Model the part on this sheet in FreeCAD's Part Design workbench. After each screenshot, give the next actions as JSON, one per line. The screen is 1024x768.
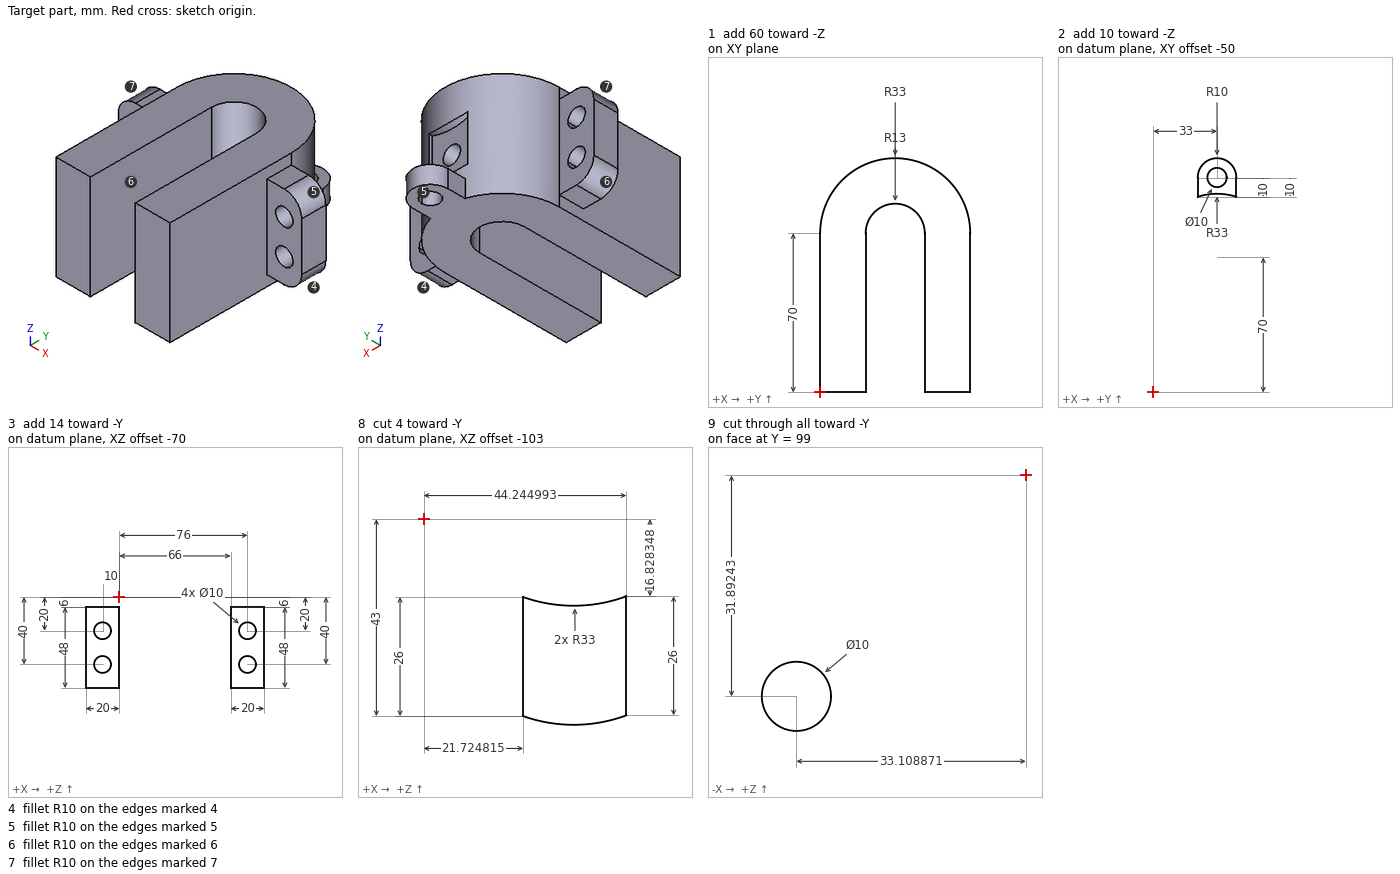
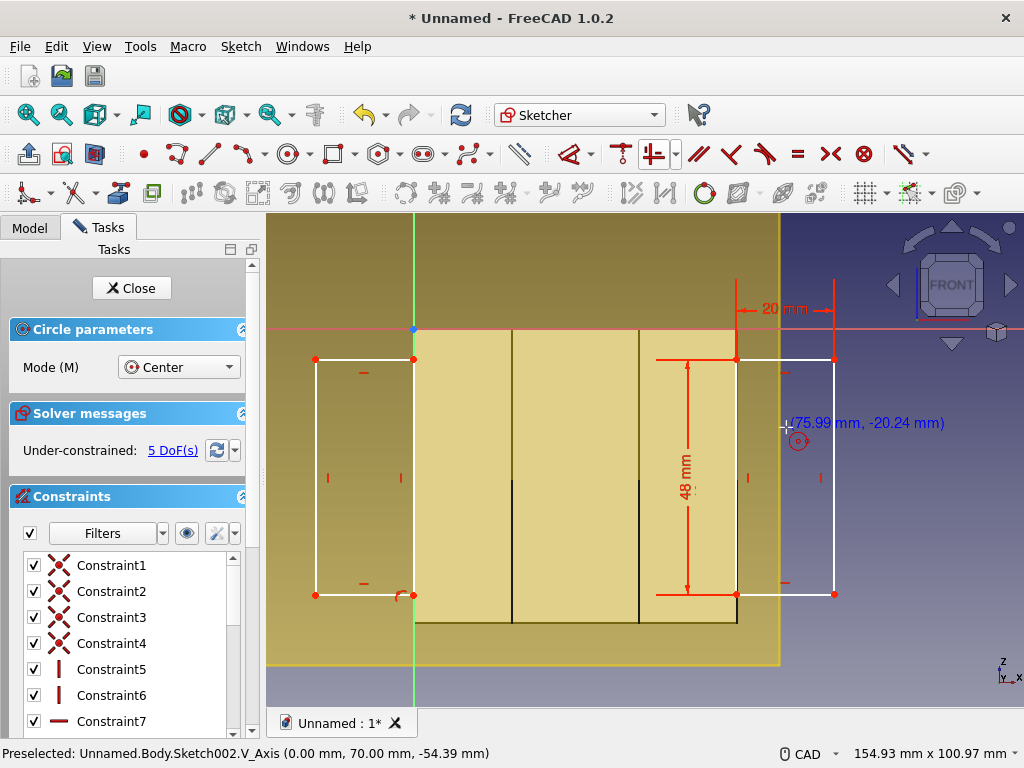
{"action": "left_click", "coordinate": [786, 427]}
{"action": "mouse_move", "coordinate": [803, 410]}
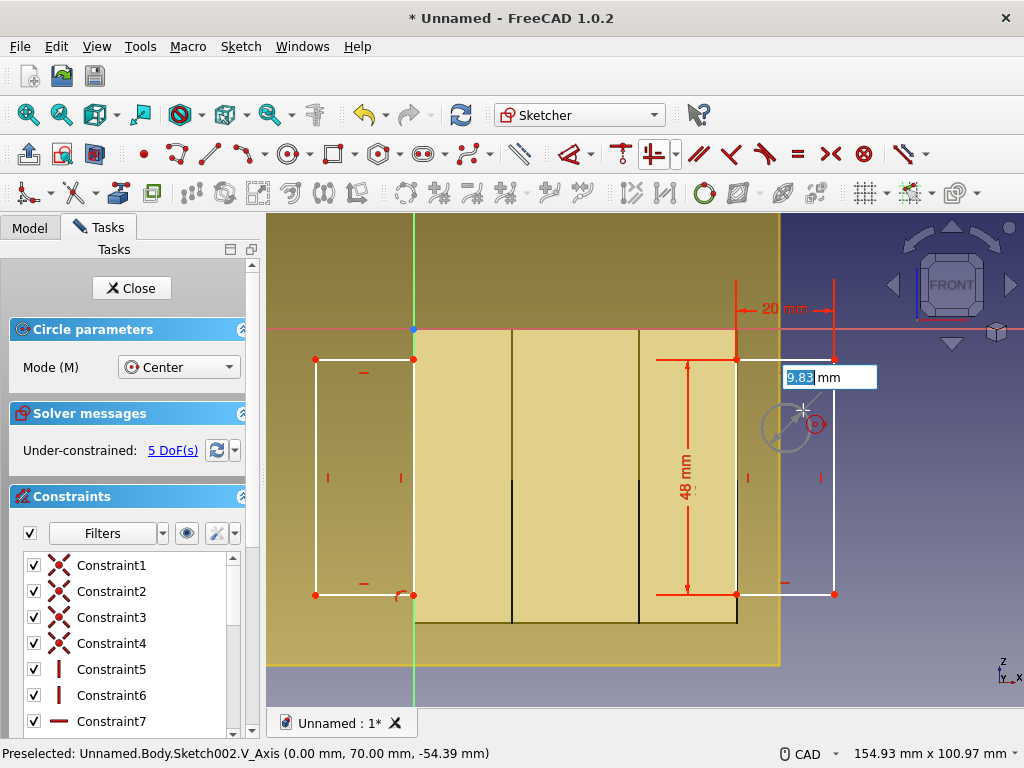
{"action": "type", "text": "10"}
{"action": "key", "text": "Return"}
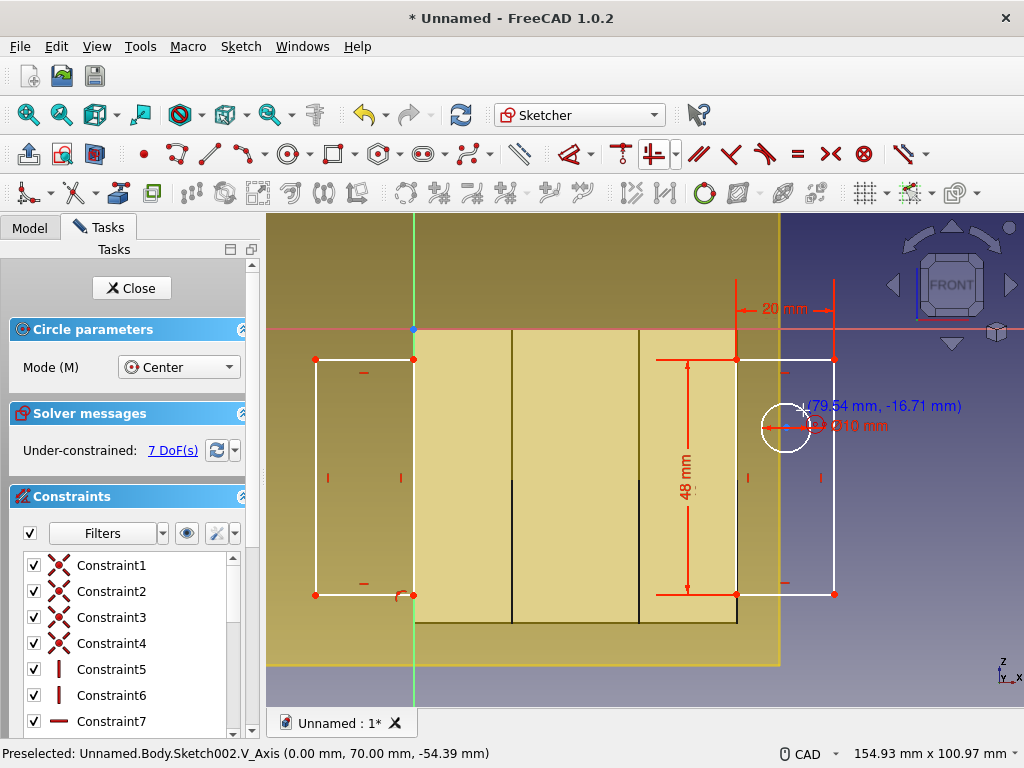
{"action": "left_click", "coordinate": [786, 525]}
{"action": "mouse_move", "coordinate": [803, 508]}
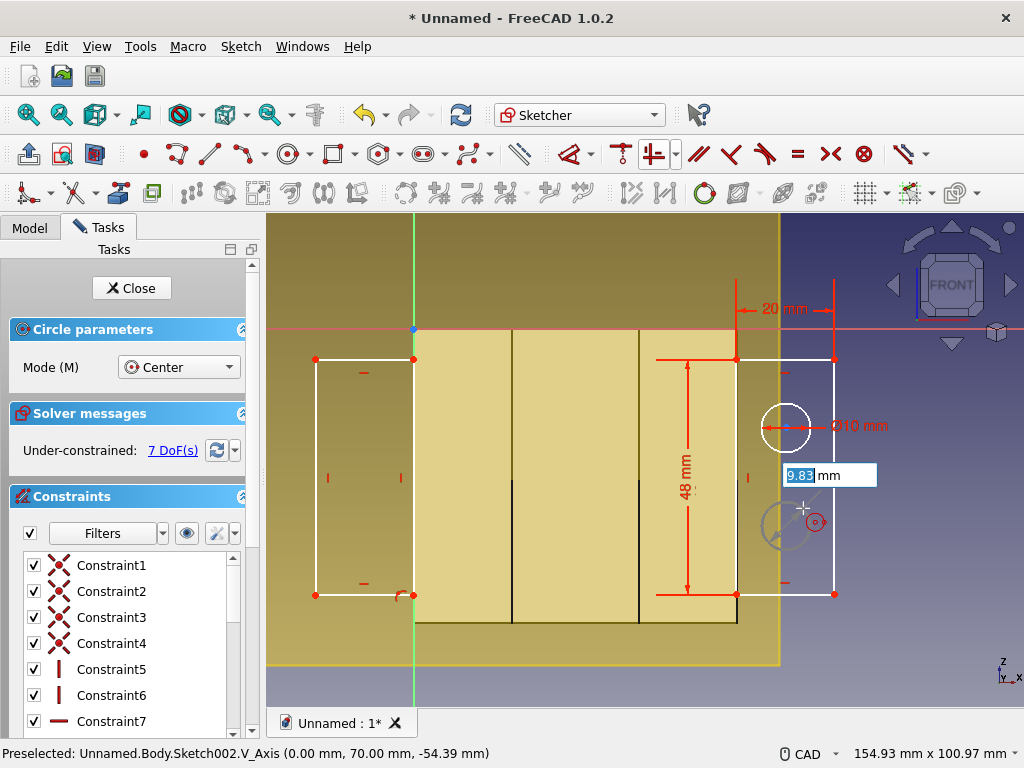
{"action": "type", "text": "10"}
{"action": "key", "text": "Return"}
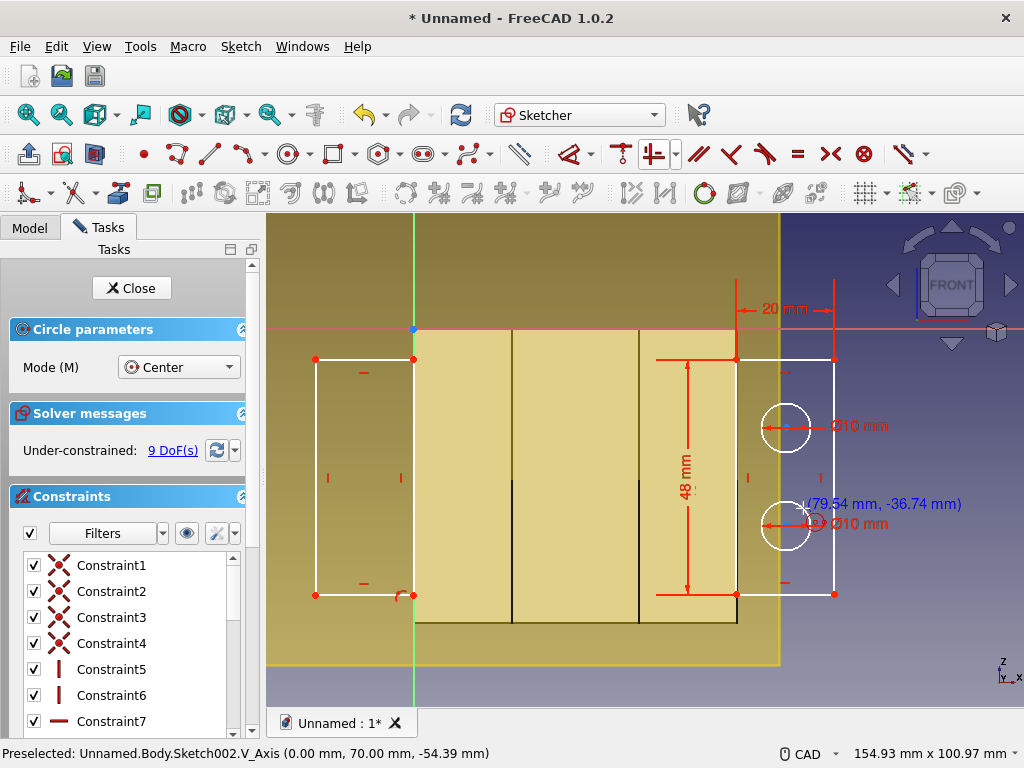
{"action": "left_click", "coordinate": [365, 427]}
{"action": "mouse_move", "coordinate": [382, 410]}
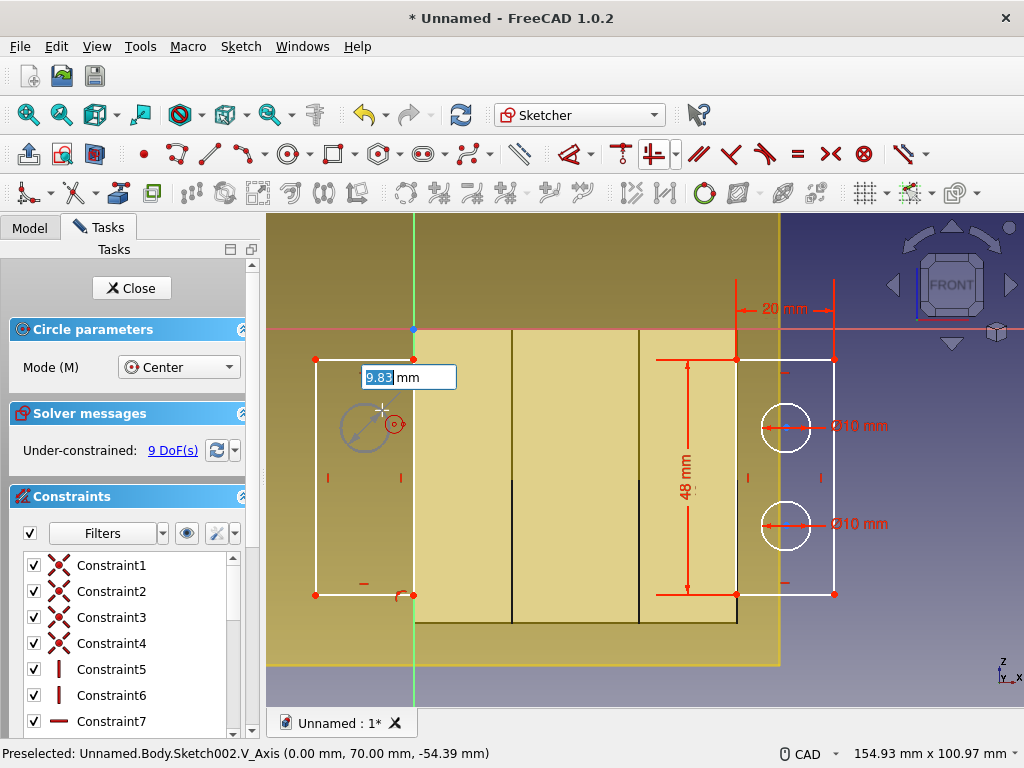
{"action": "type", "text": "10"}
{"action": "key", "text": "Return"}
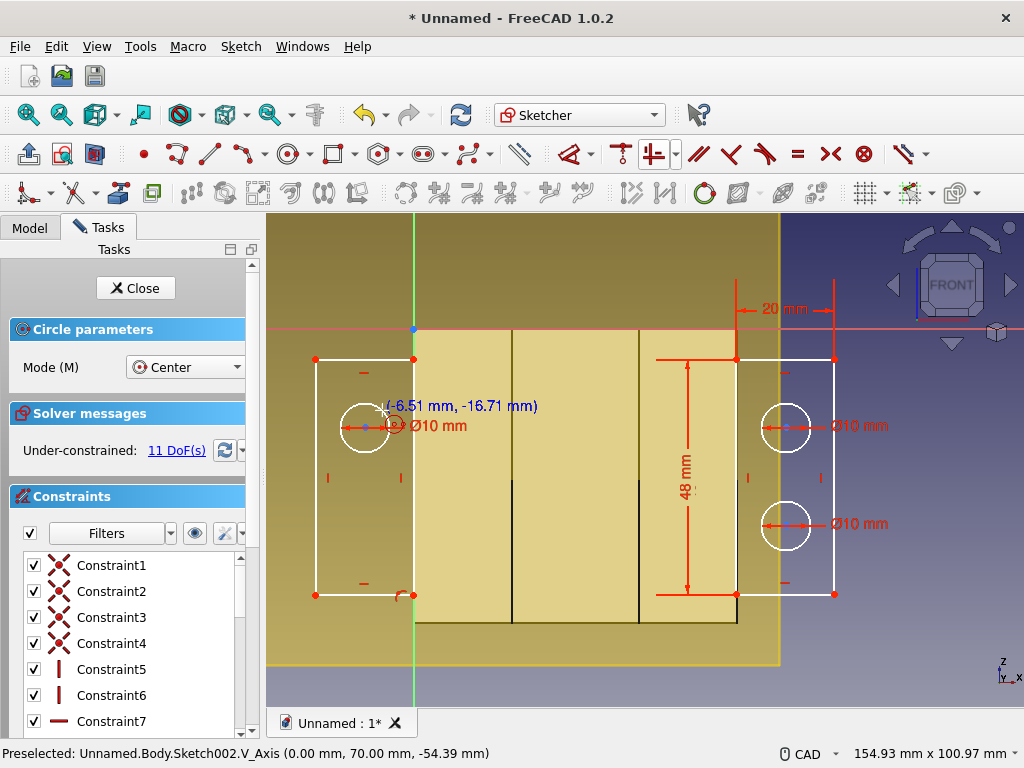
{"action": "left_click", "coordinate": [365, 525]}
{"action": "mouse_move", "coordinate": [382, 508]}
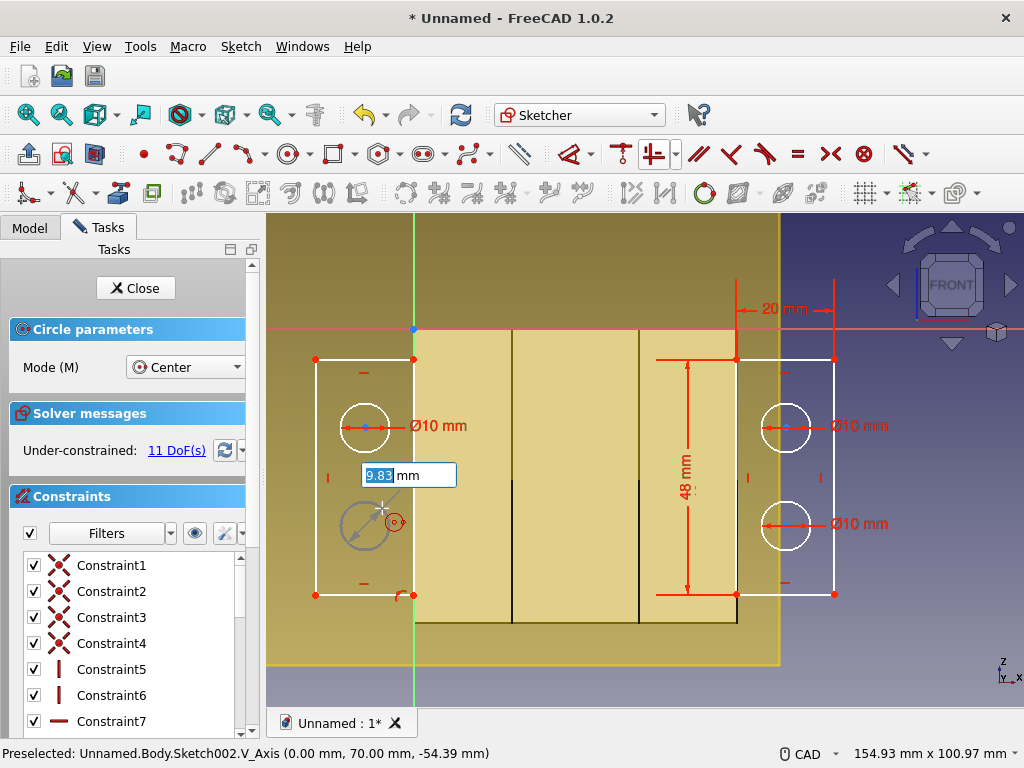
{"action": "type", "text": "10"}
{"action": "key", "text": "Return"}
{"action": "key", "text": "Escape"}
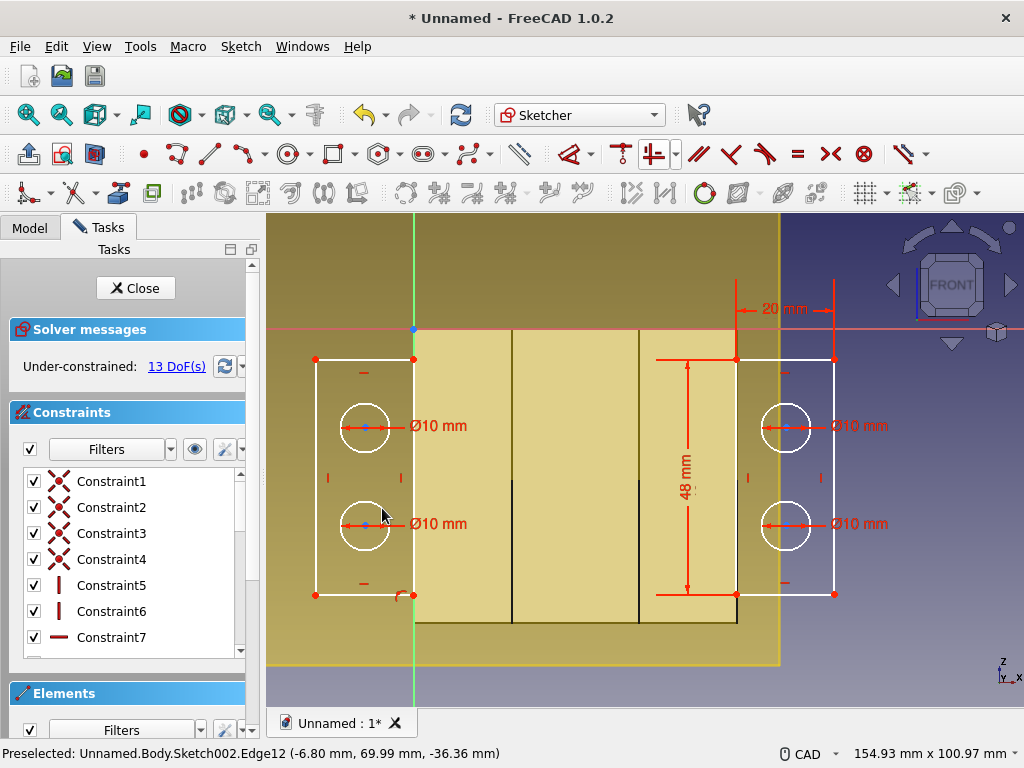
{"action": "left_click", "coordinate": [786, 428]}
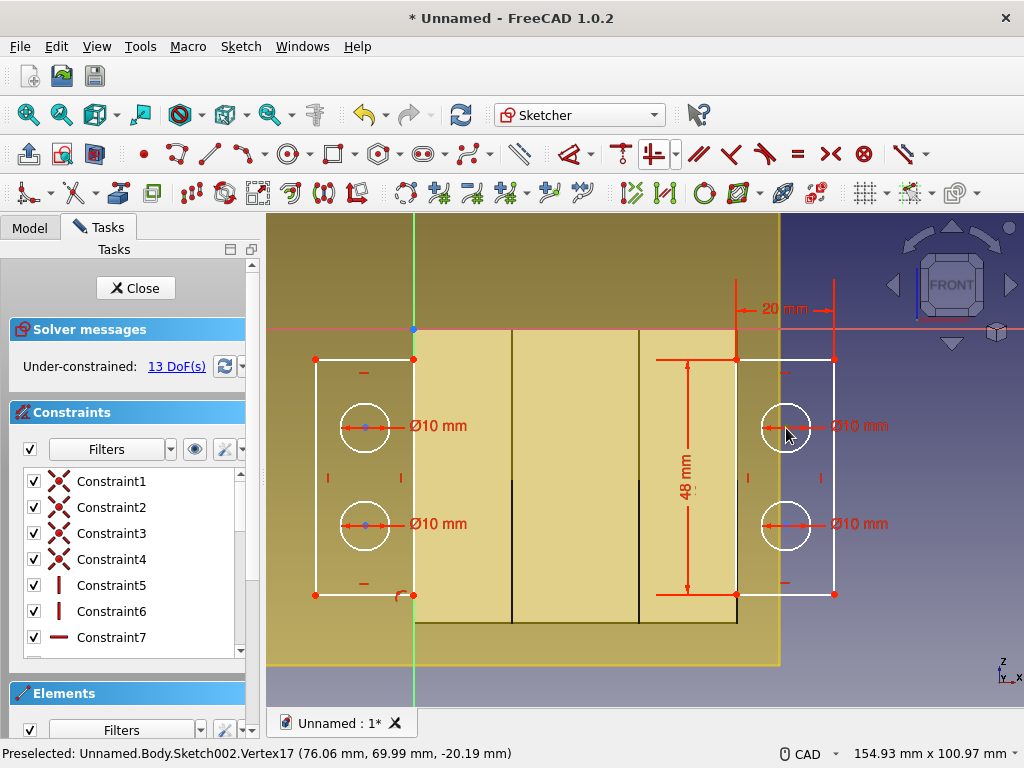
{"action": "left_click", "coordinate": [786, 526]}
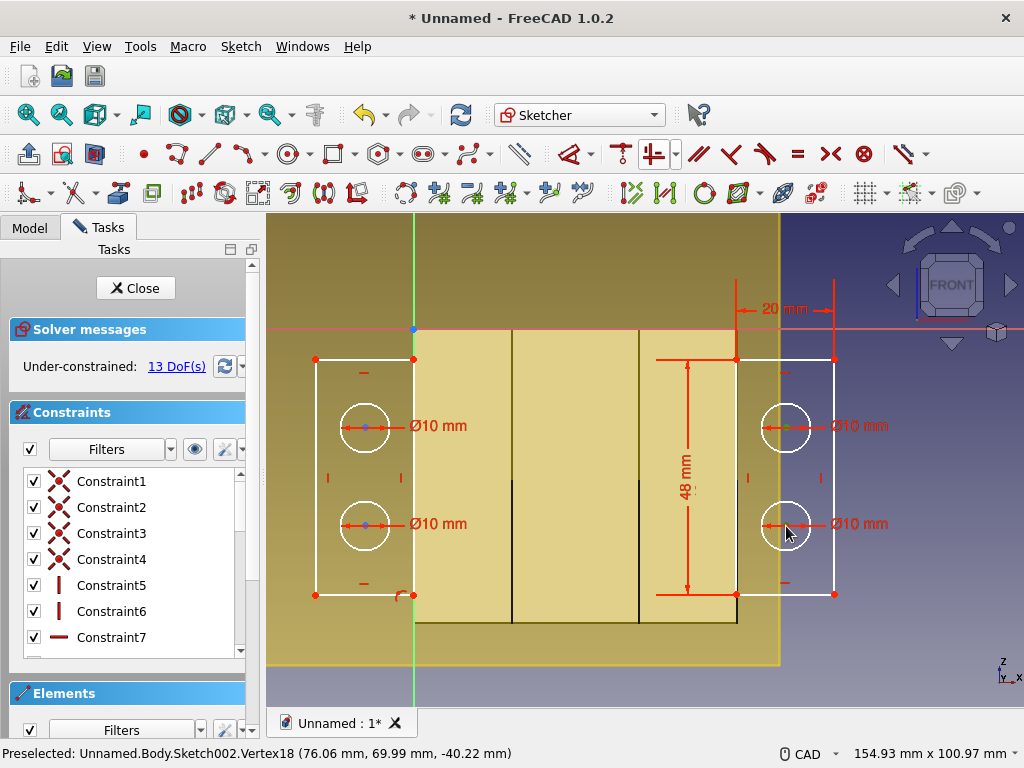
{"action": "key", "text": "v"}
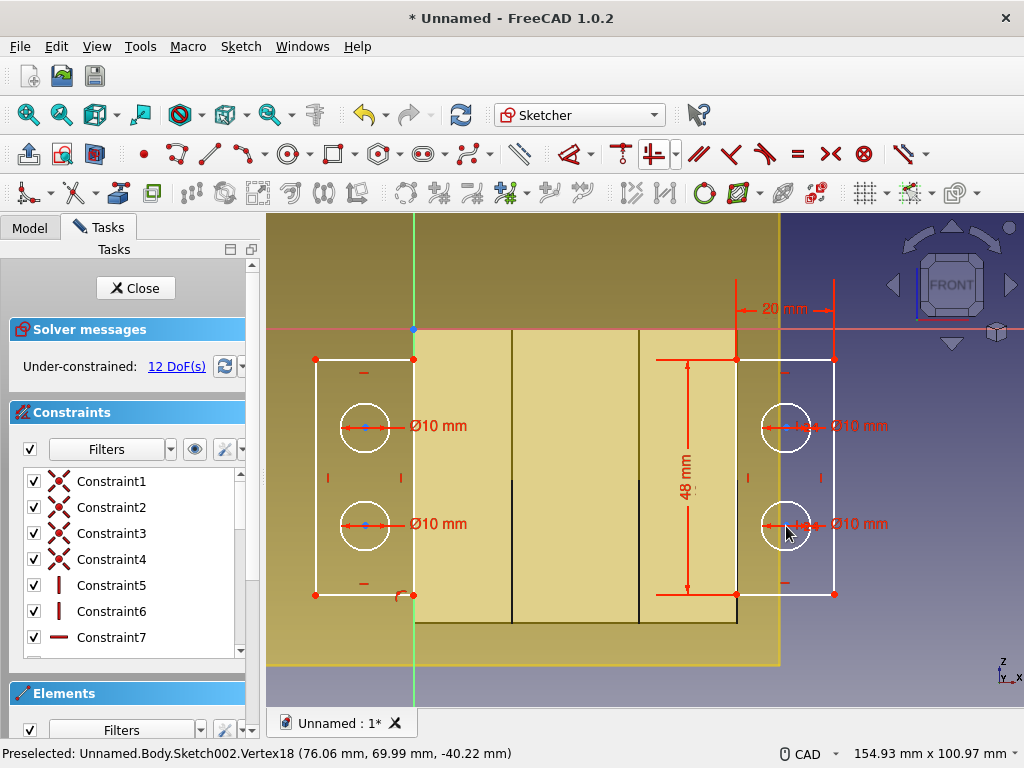
{"action": "left_click", "coordinate": [365, 428]}